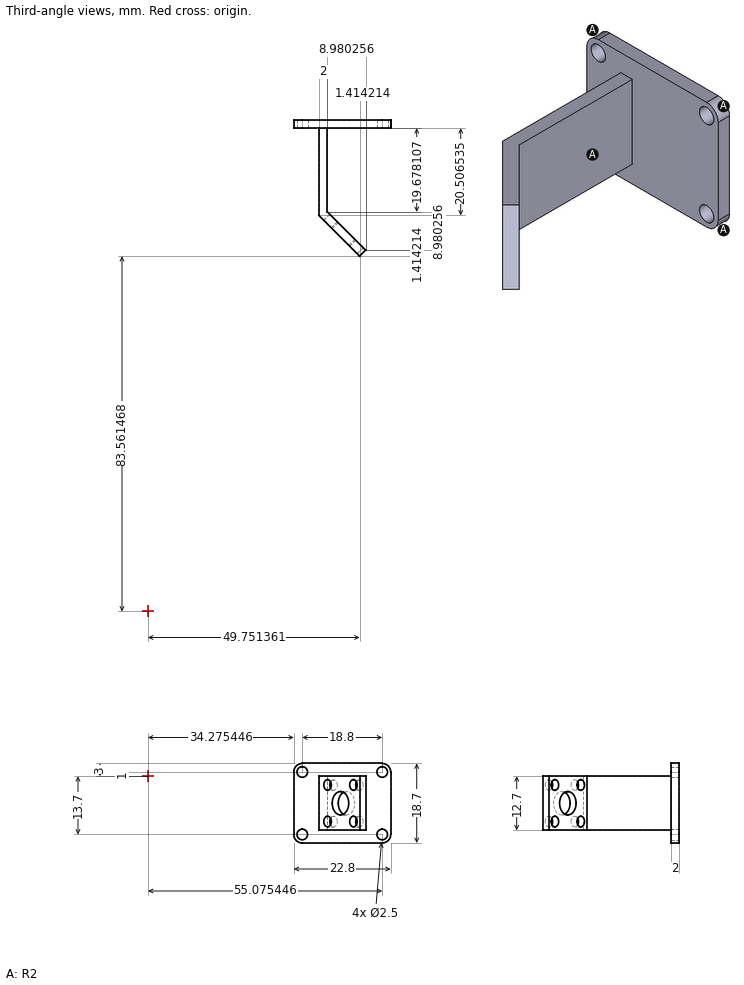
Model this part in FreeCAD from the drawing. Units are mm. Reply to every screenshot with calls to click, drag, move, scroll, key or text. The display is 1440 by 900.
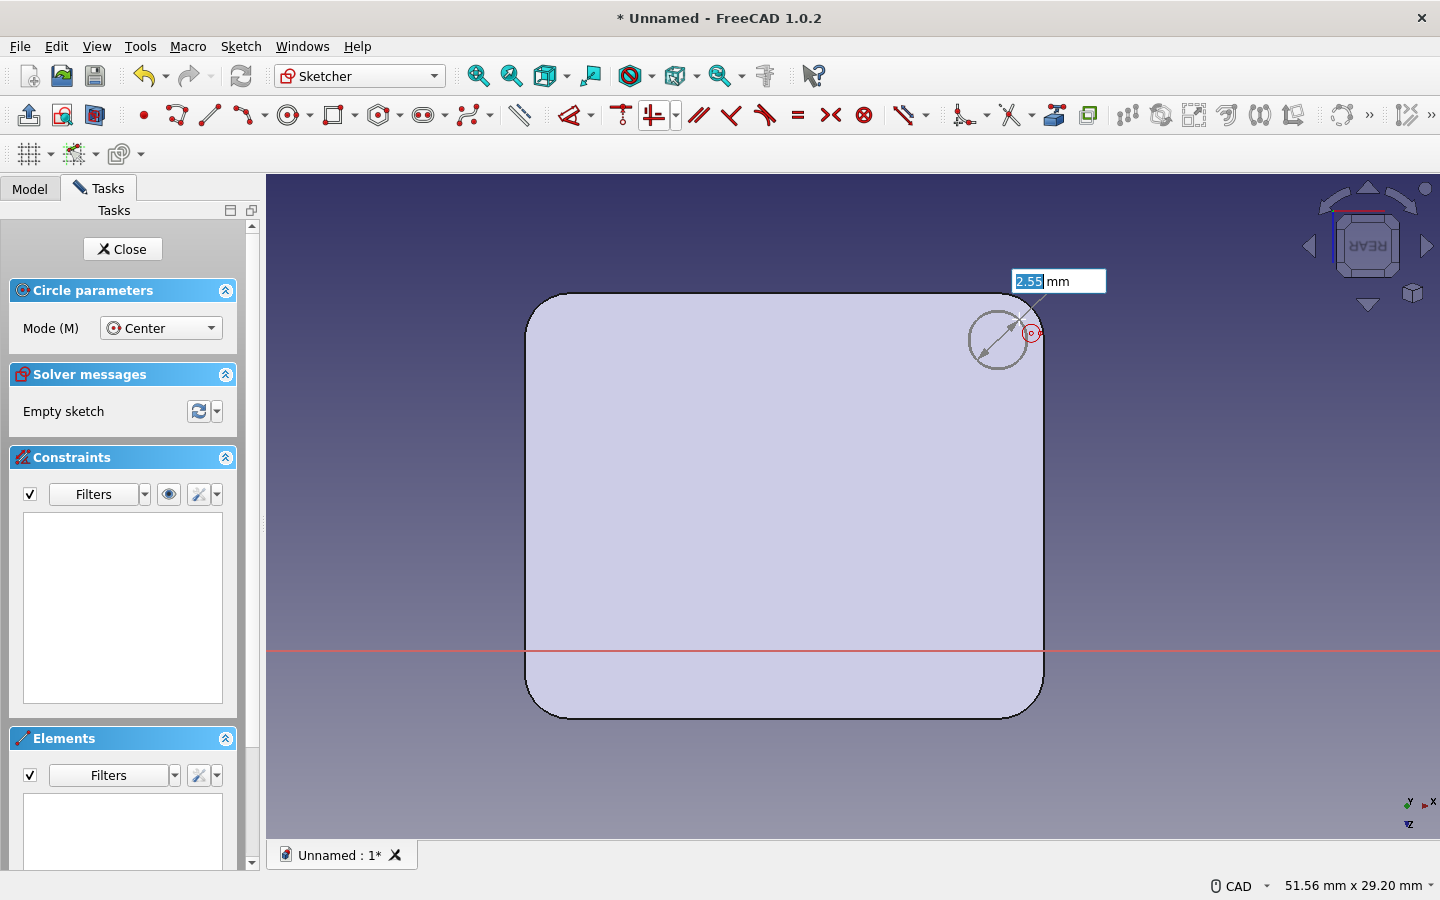
text(2.5)
key(Return)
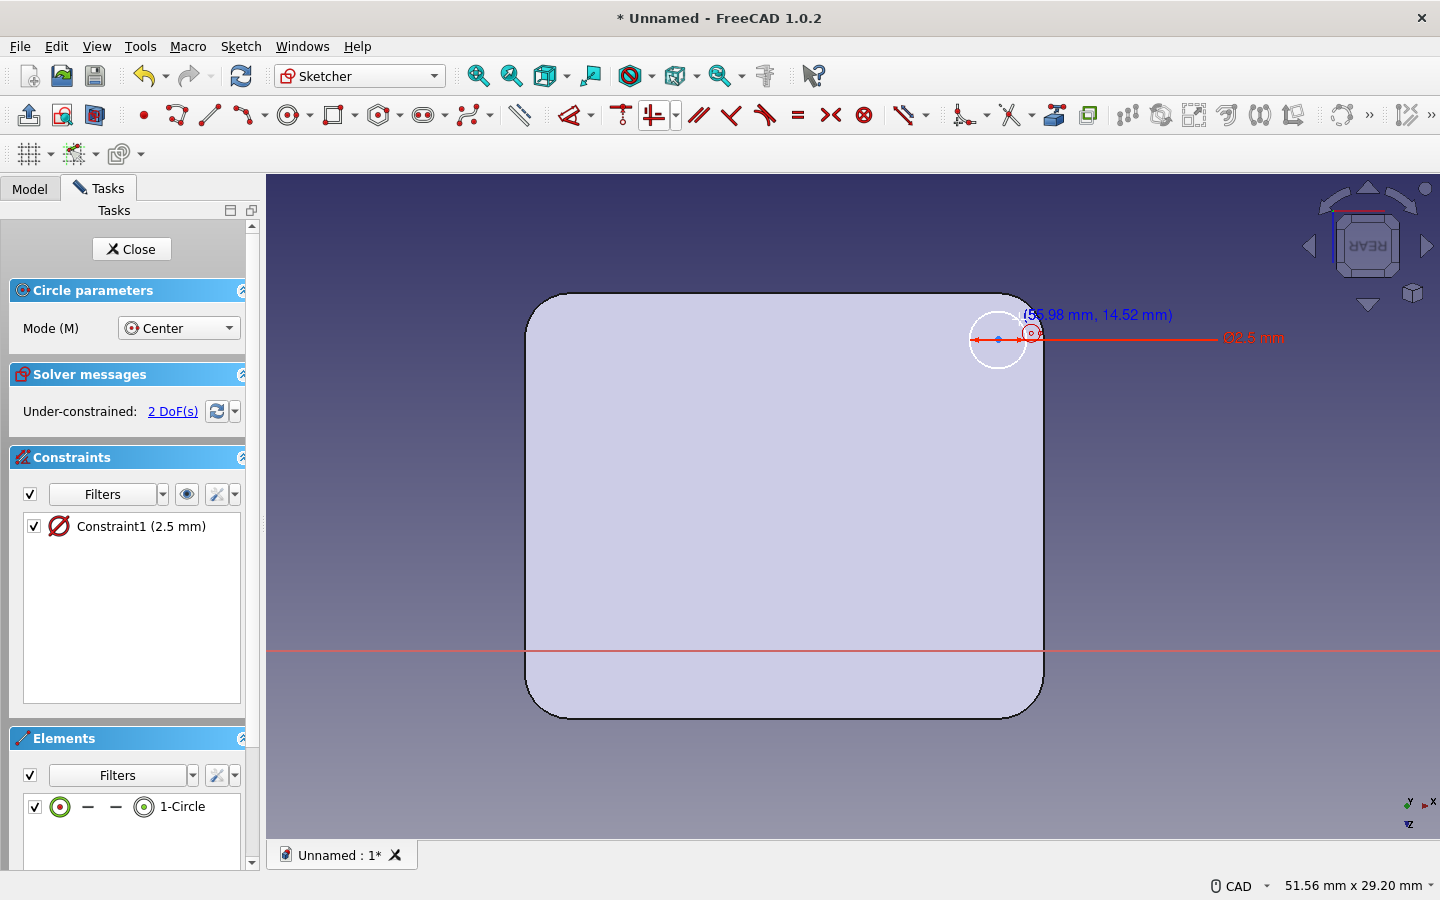
click(998, 673)
move(1019, 693)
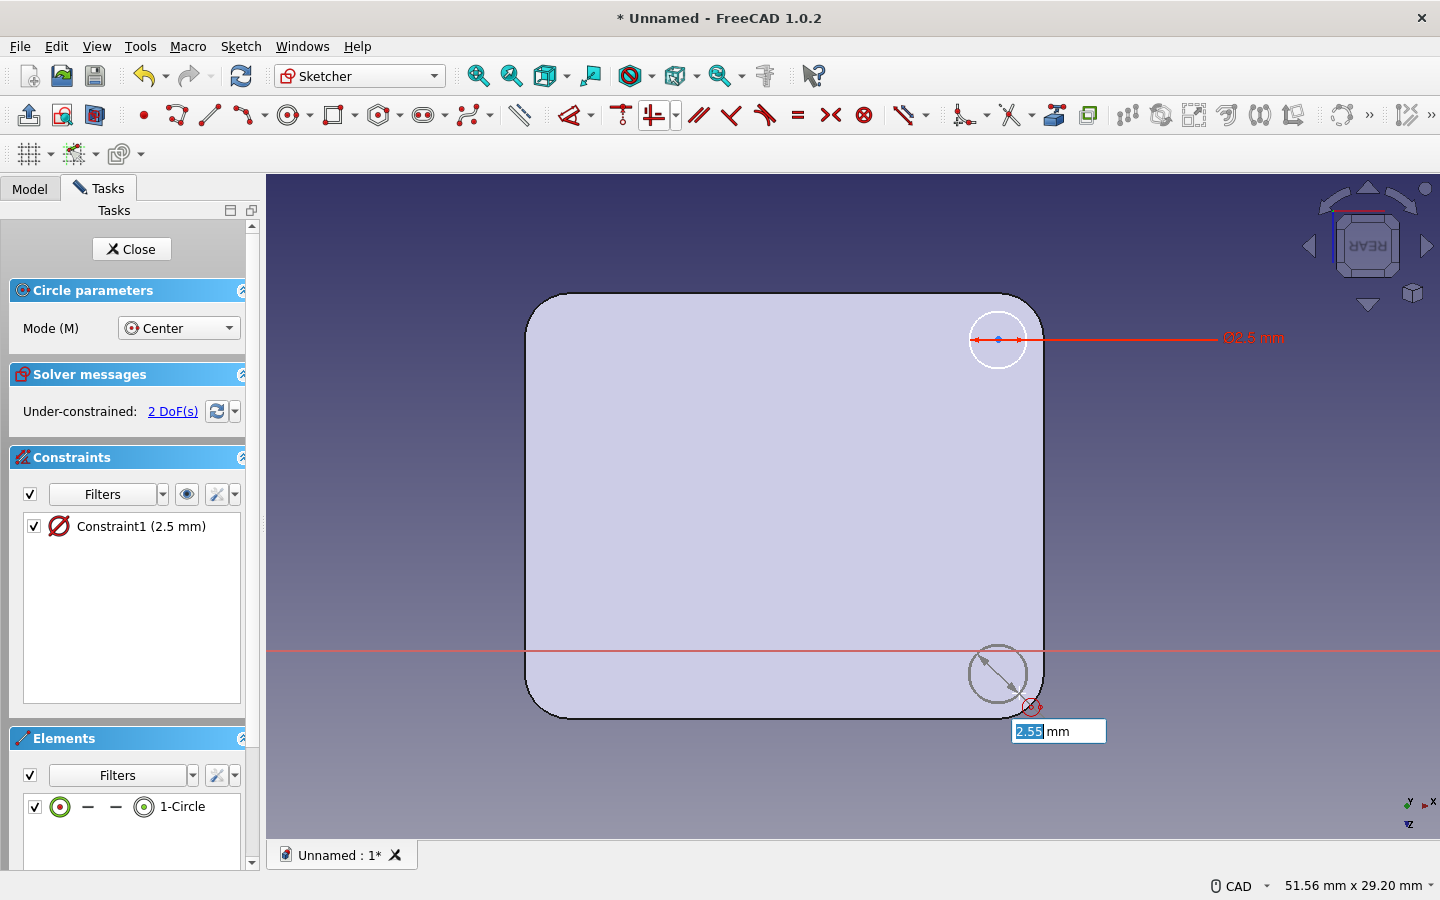
text(2.5)
key(Return)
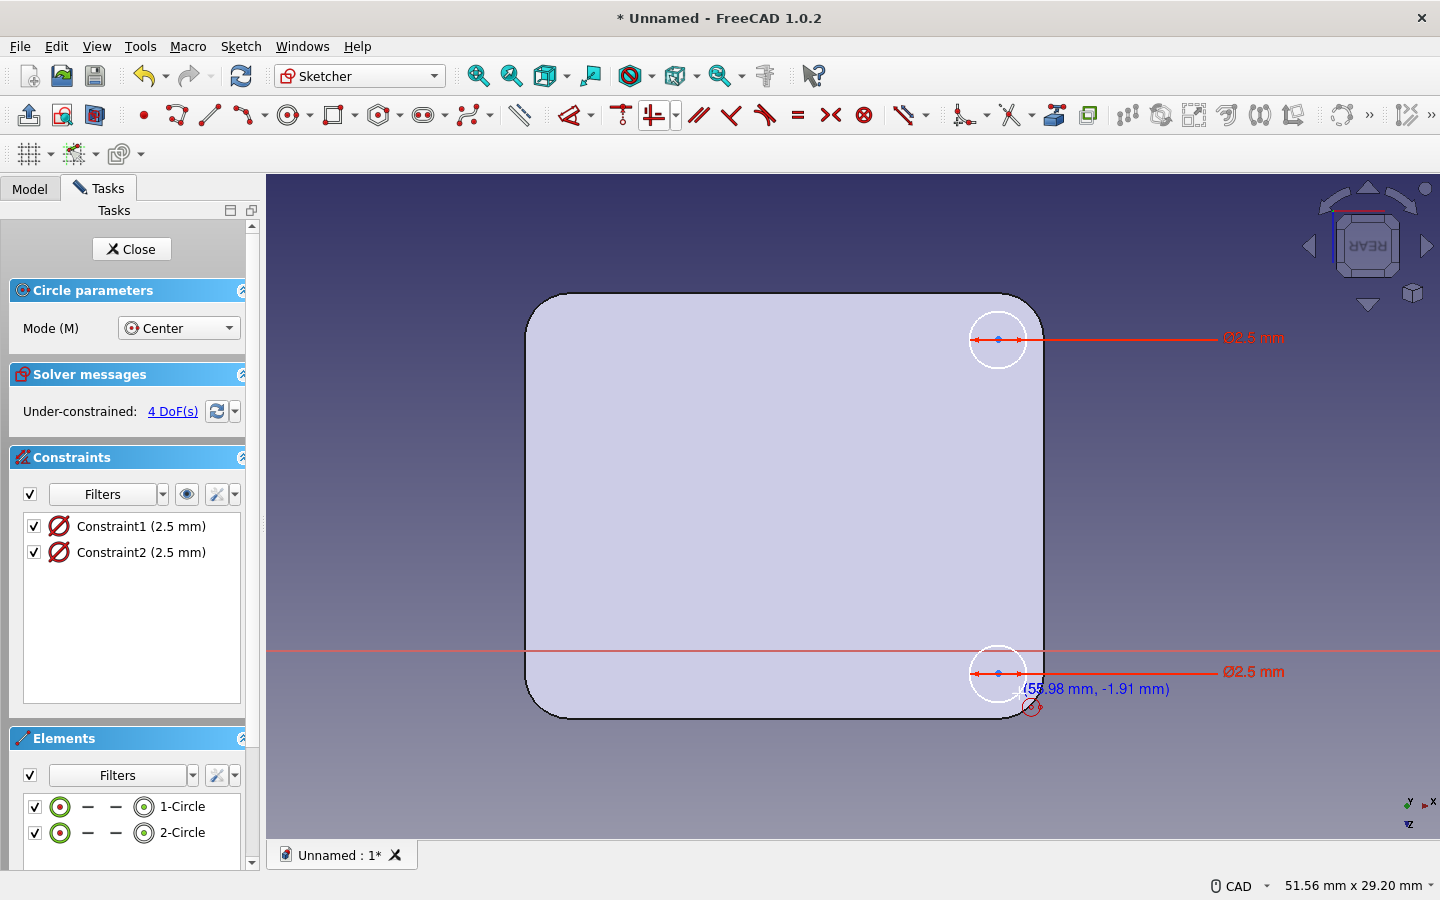
click(570, 673)
move(590, 693)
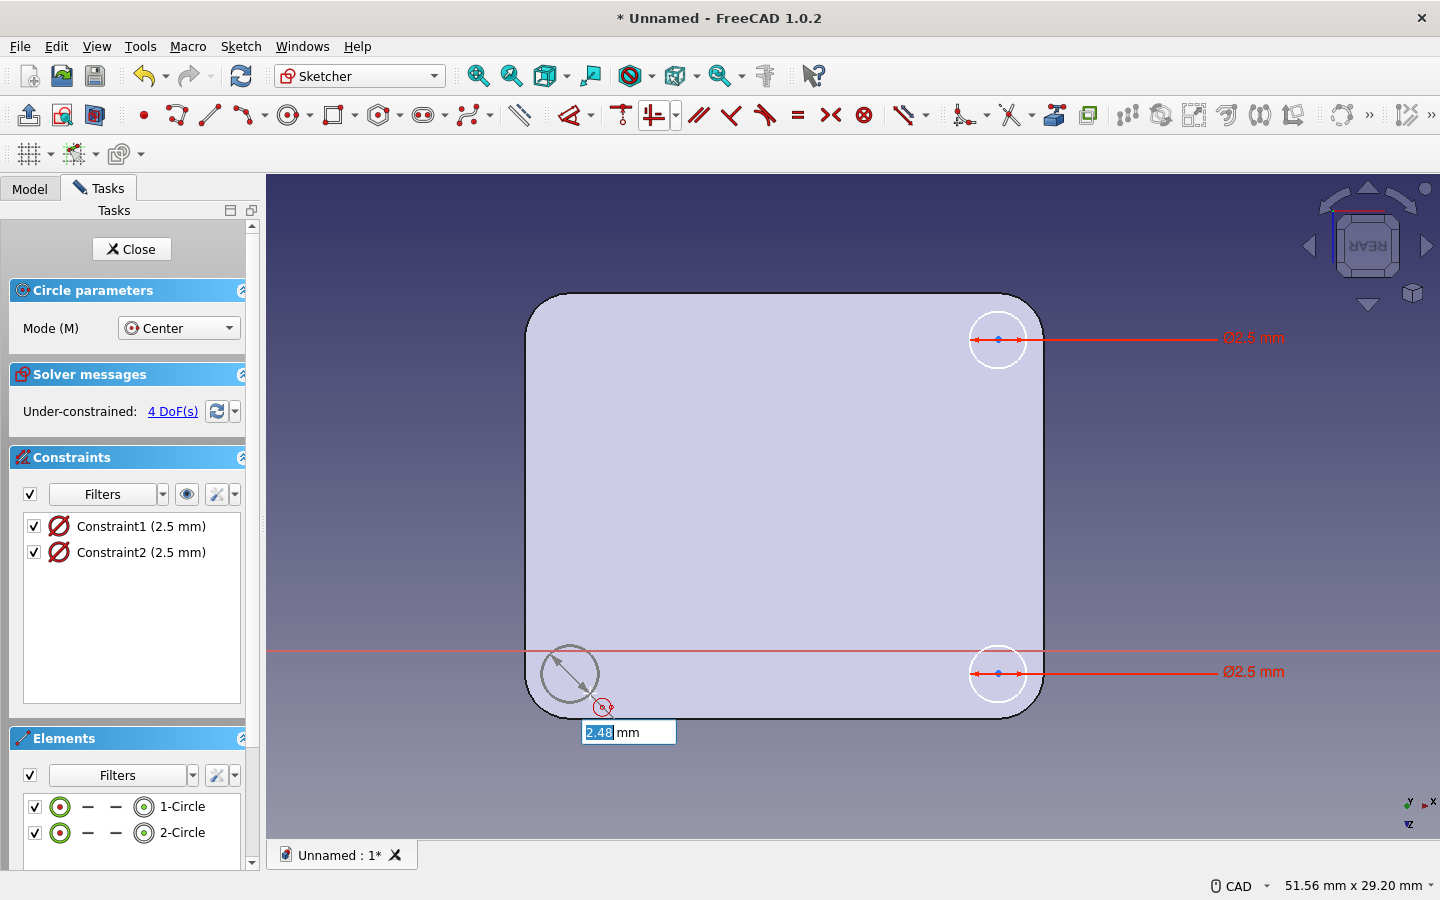
text(2.5)
key(Return)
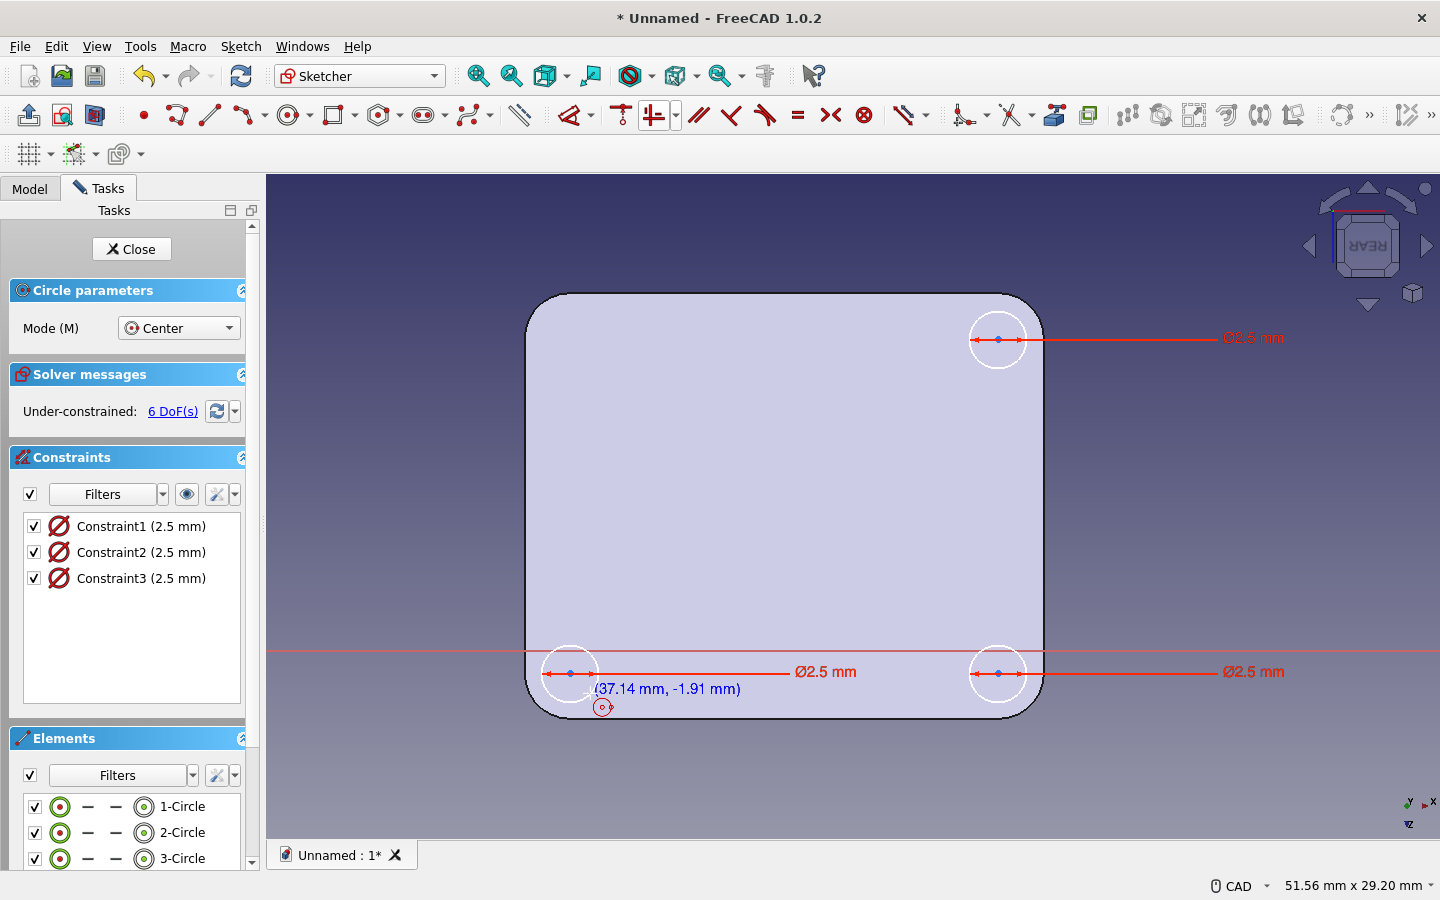
click(570, 339)
move(590, 319)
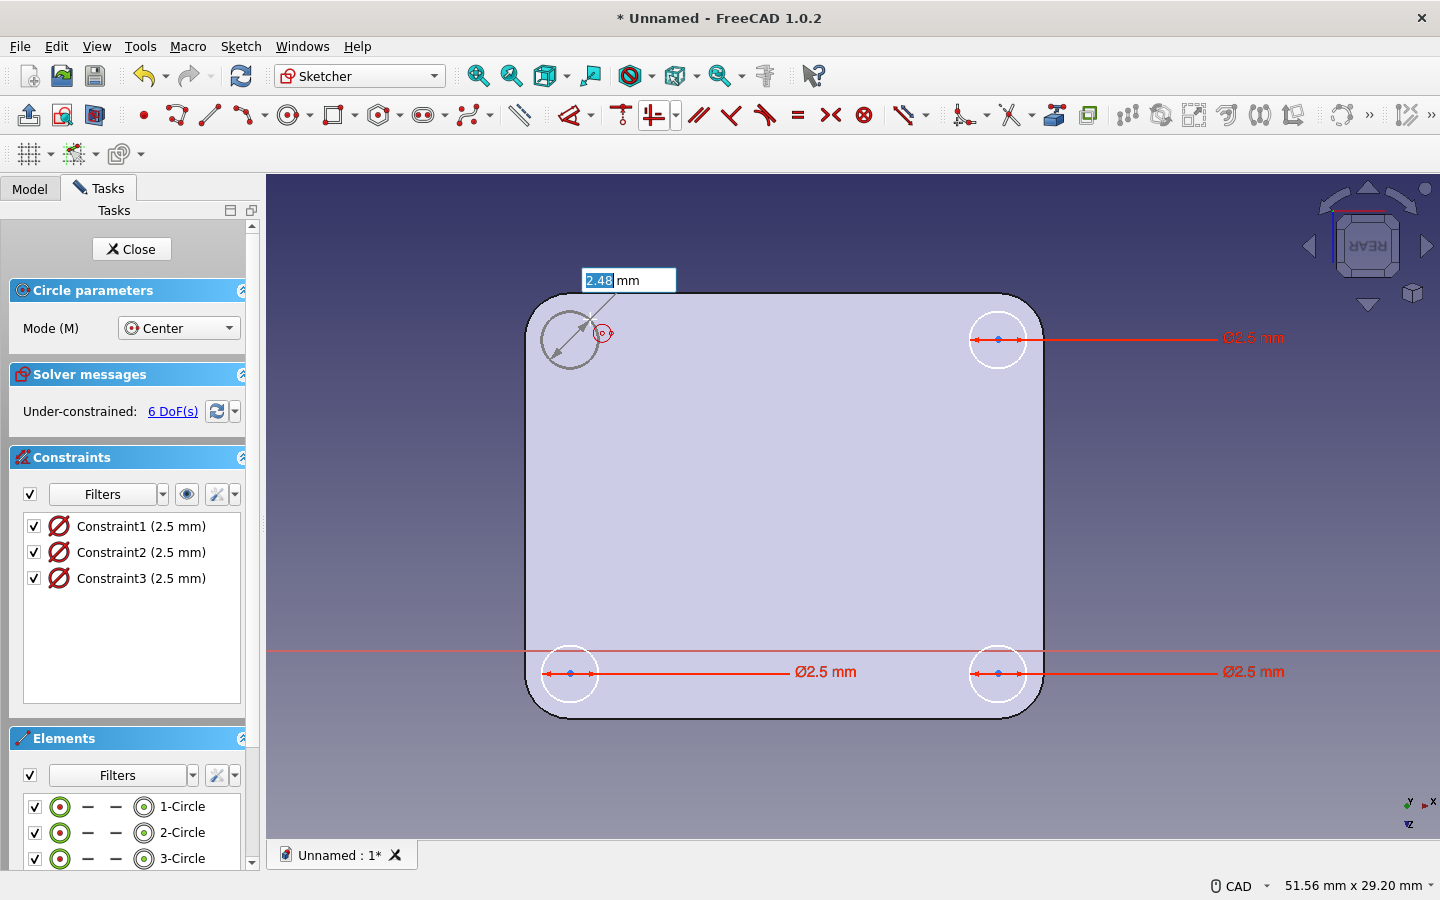
text(2.5)
key(Return)
key(Escape)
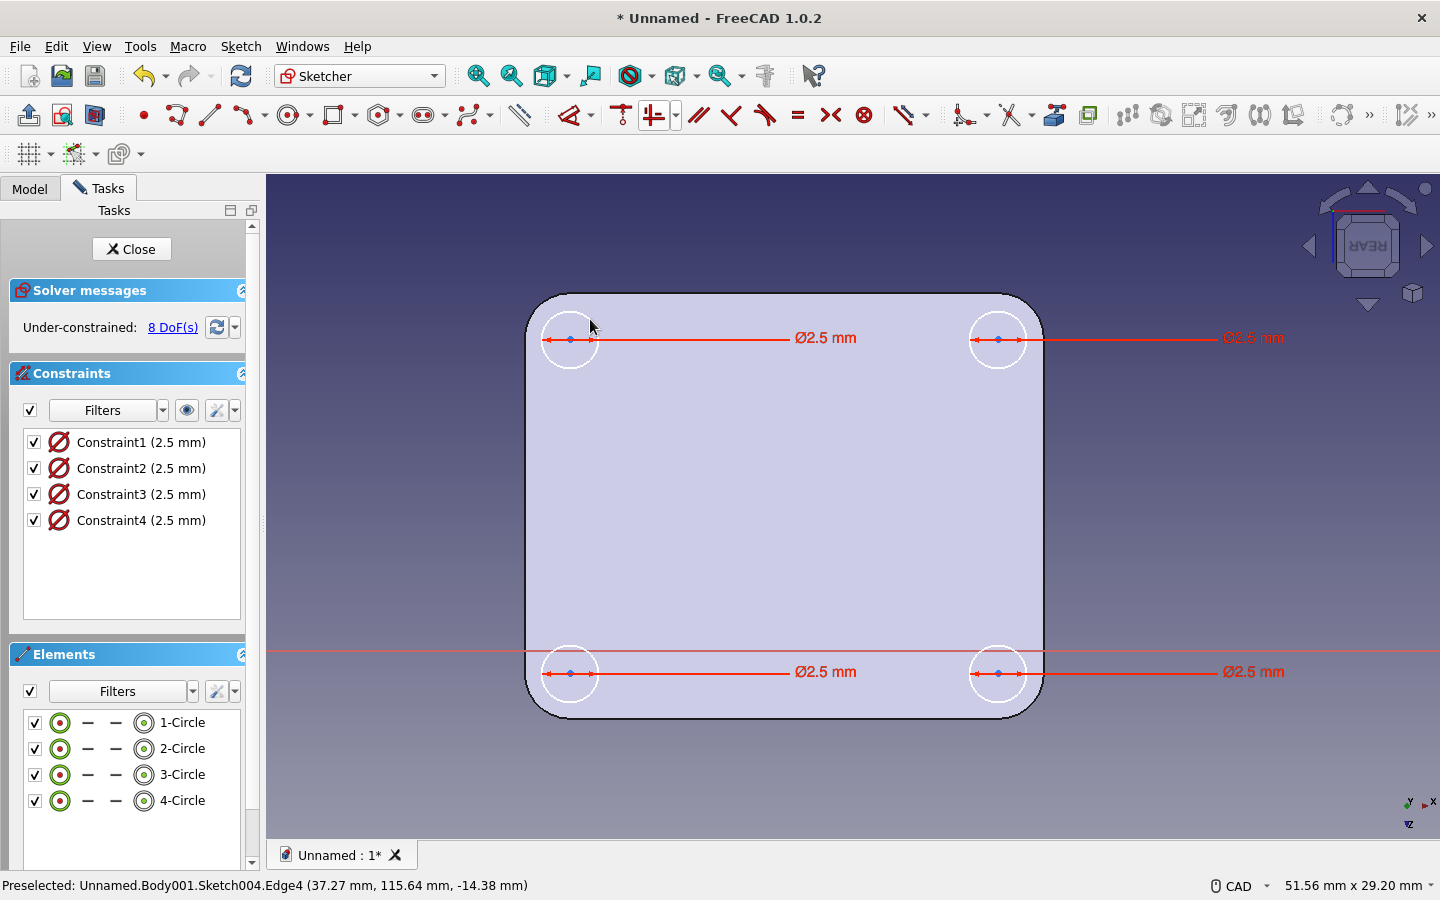
click(568, 116)